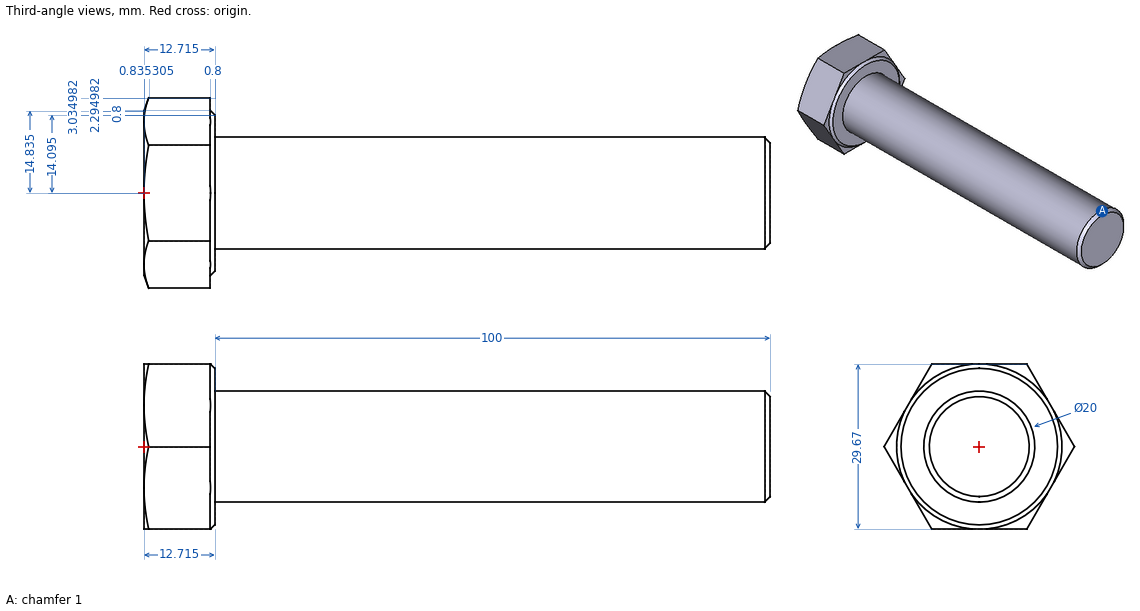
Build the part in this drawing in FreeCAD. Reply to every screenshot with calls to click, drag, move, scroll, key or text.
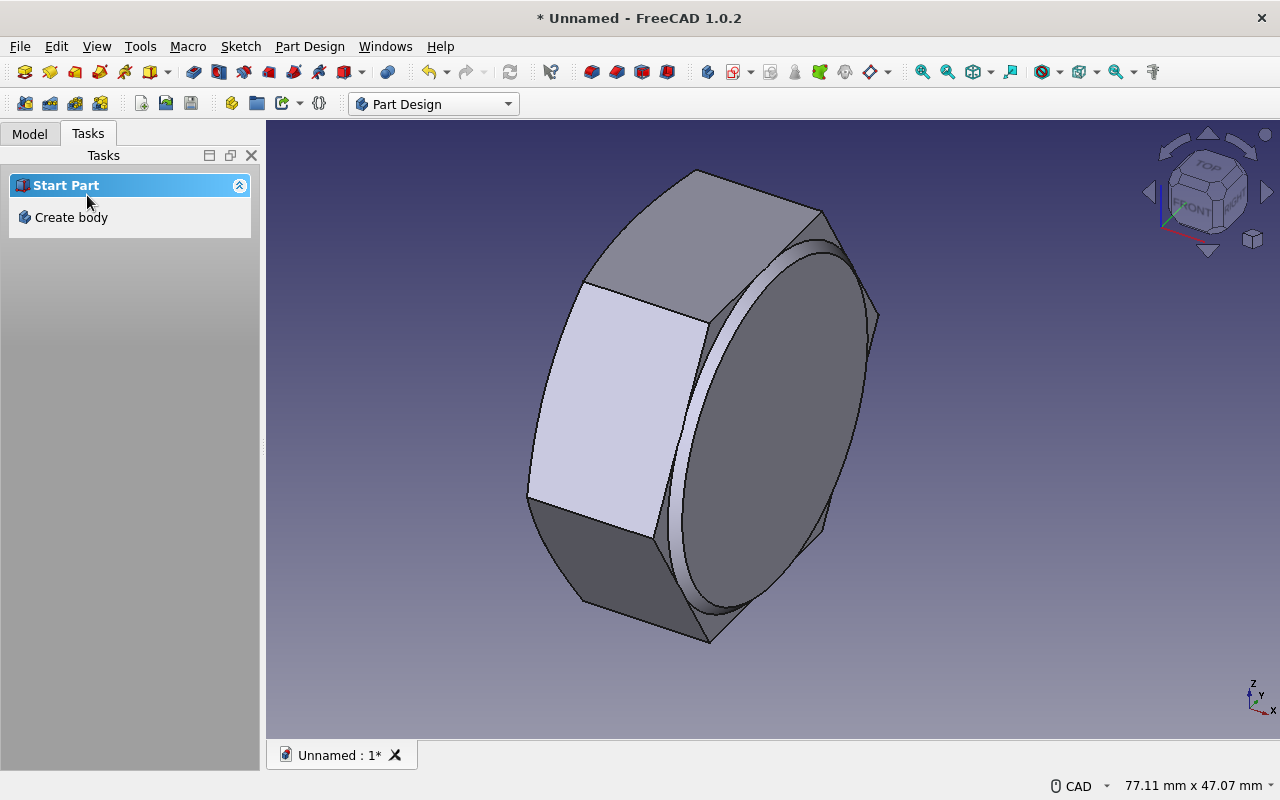
key(v)
key(f)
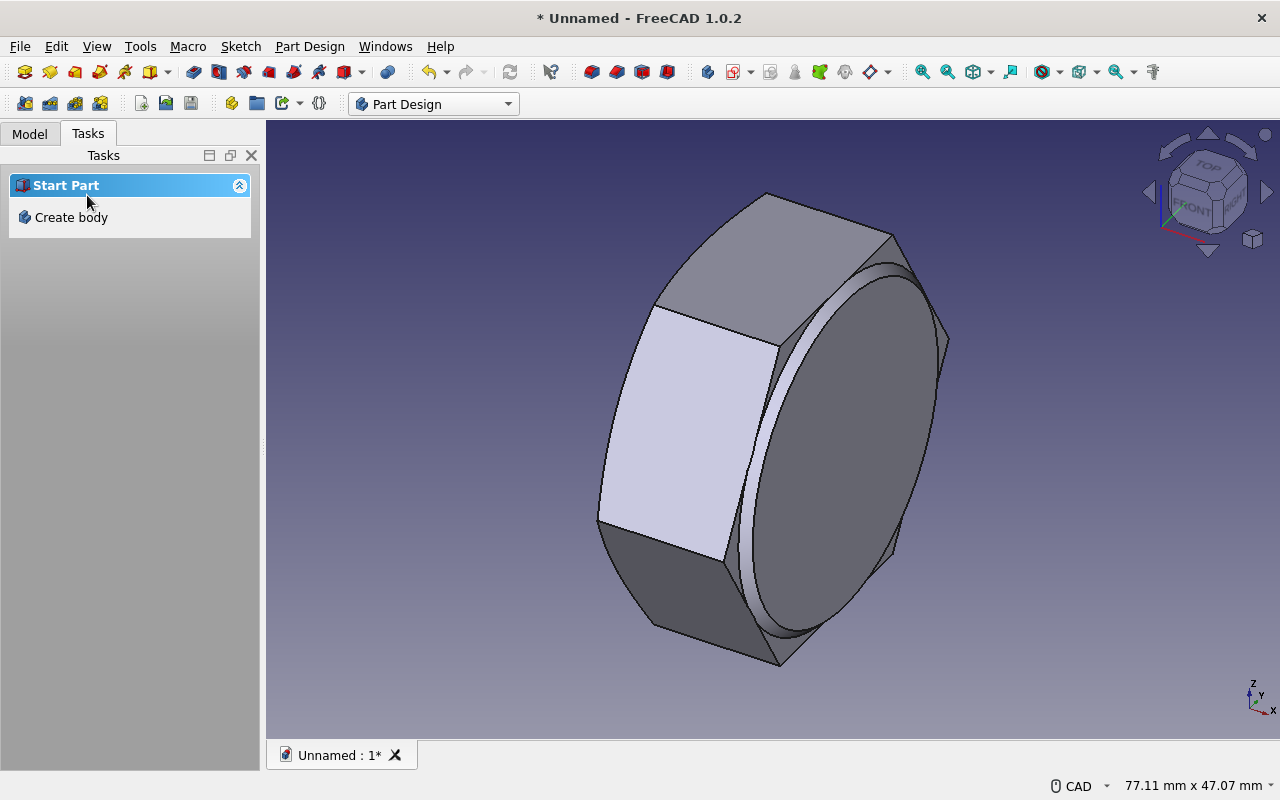
click(845, 452)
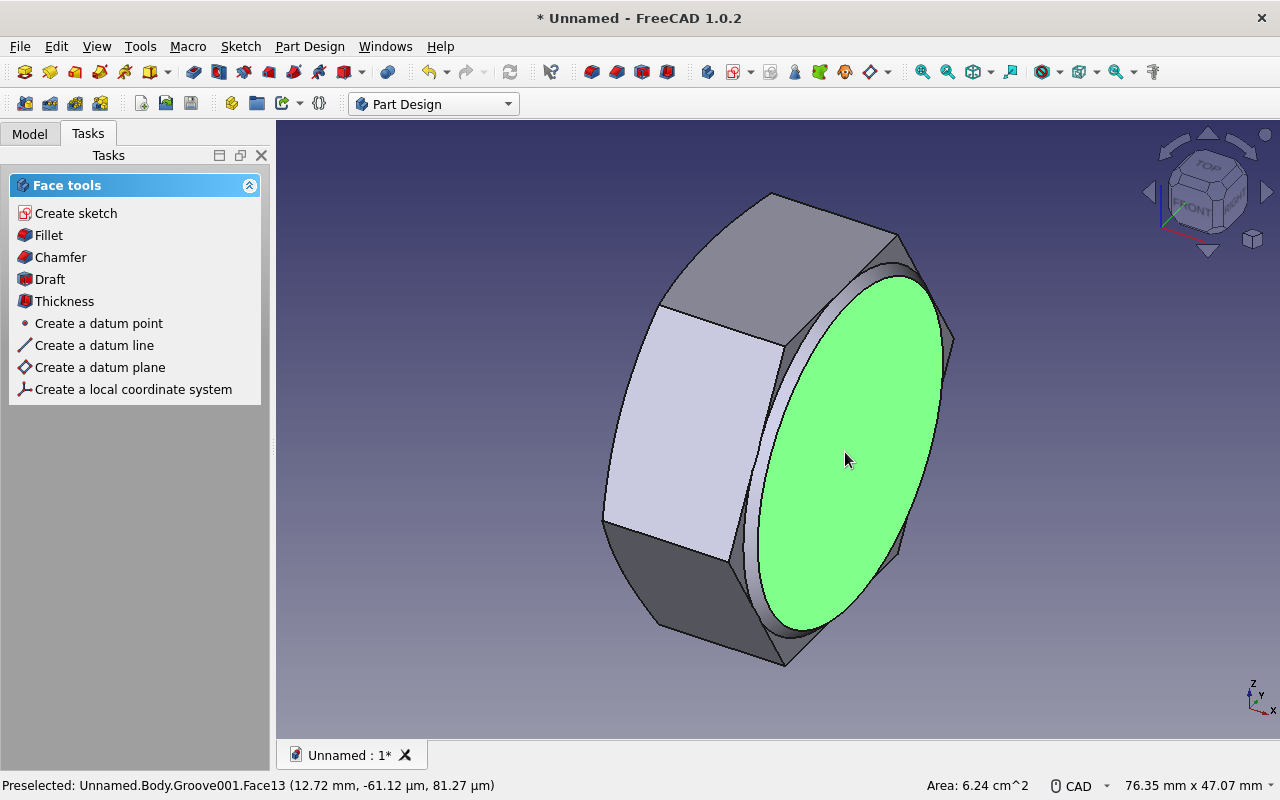
click(732, 72)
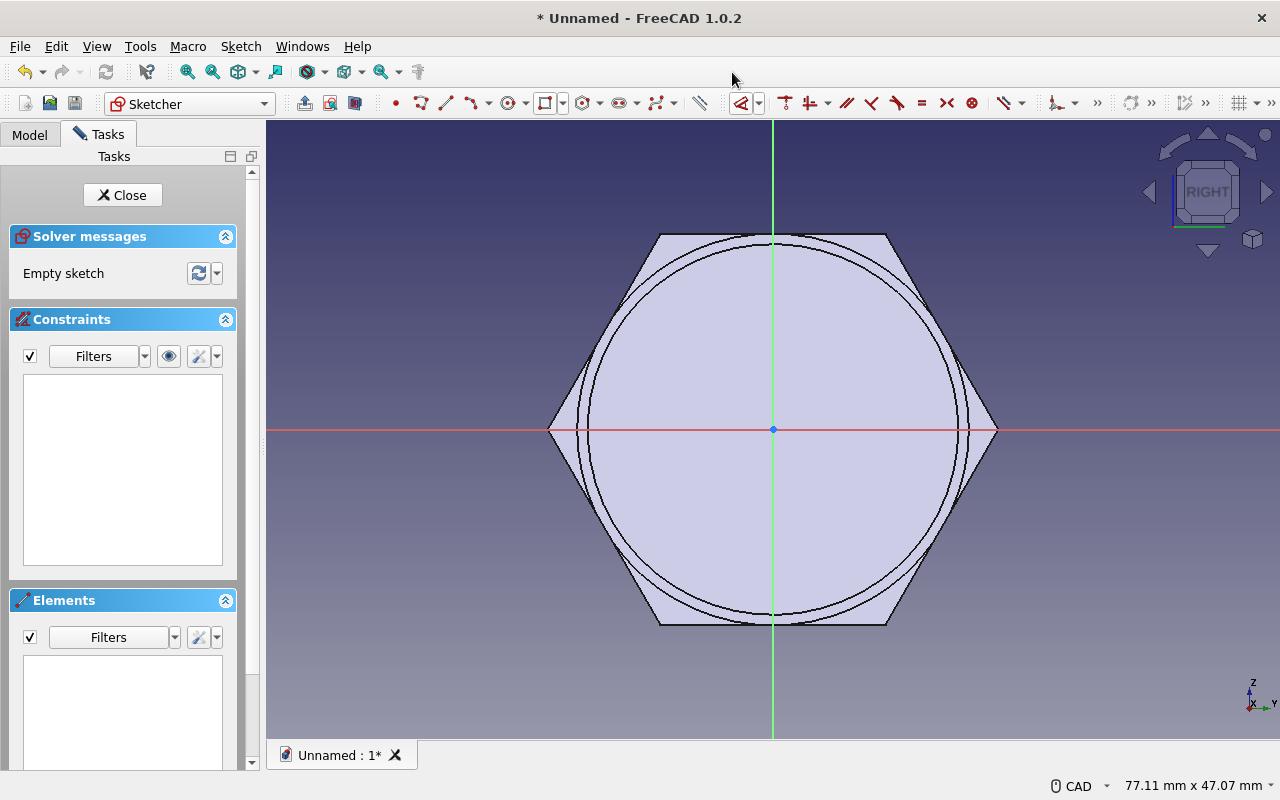
scroll(912, 429, up, 2)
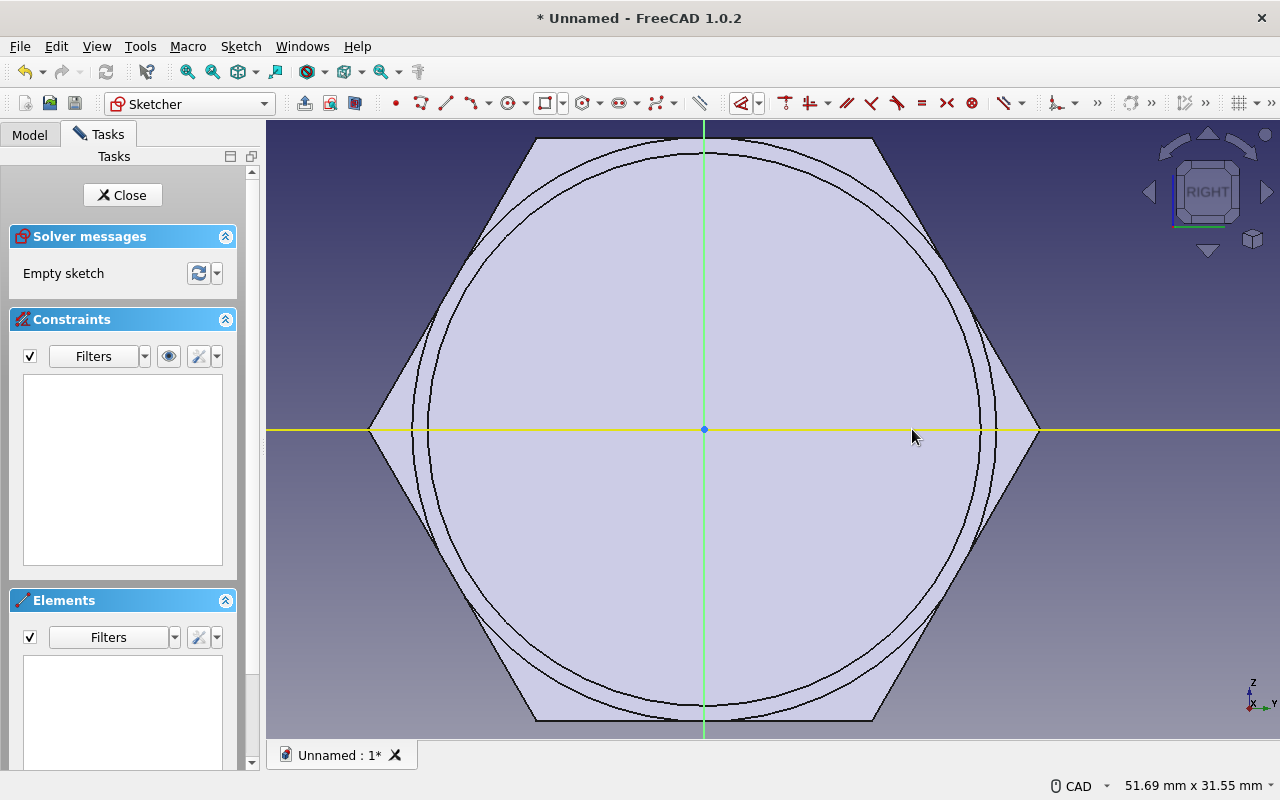
key(g)
key(c)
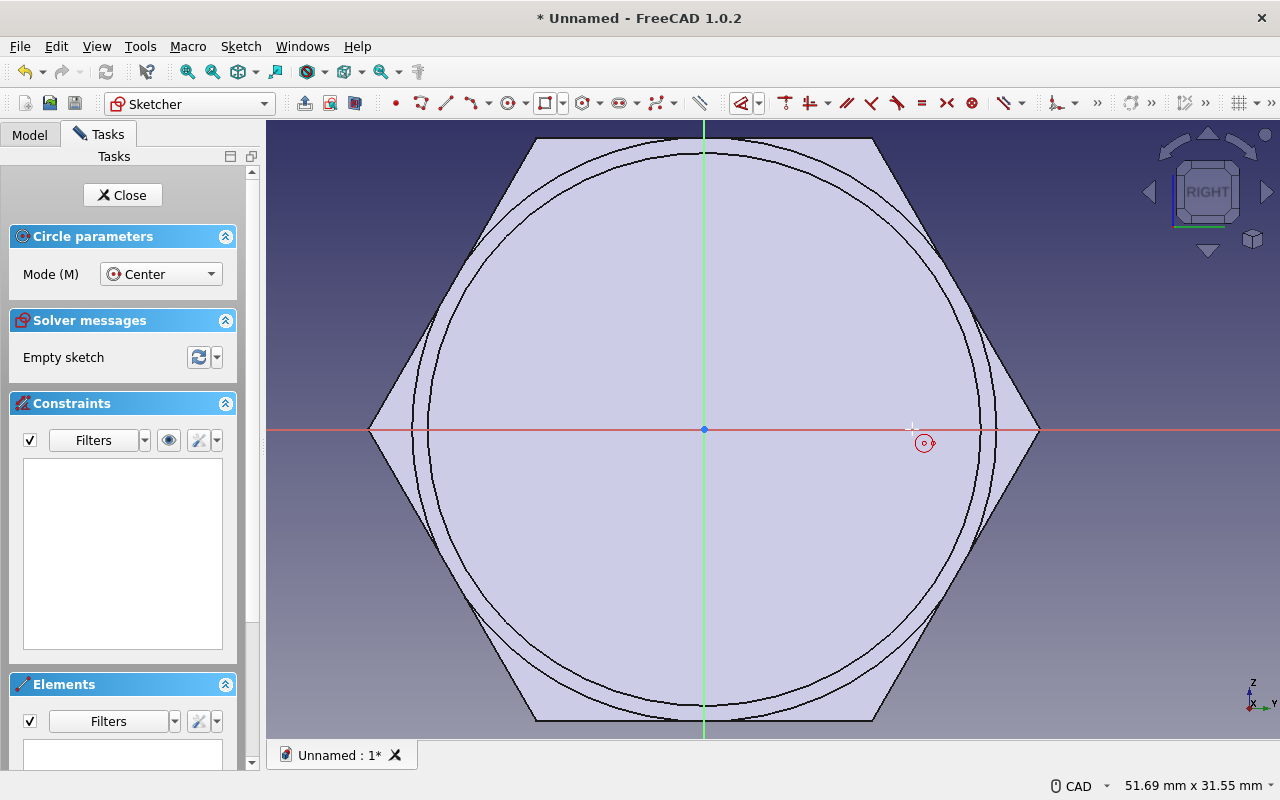
click(704, 429)
move(843, 291)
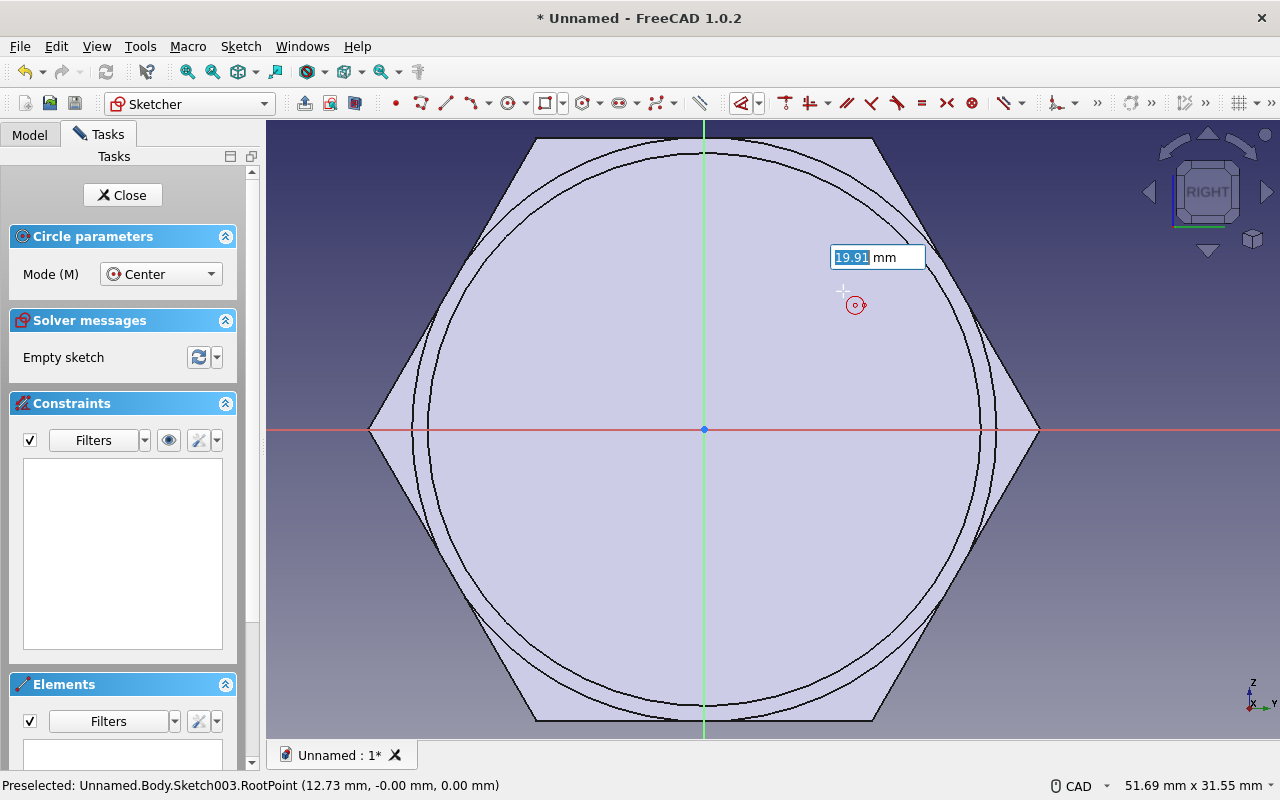
text(20)
key(Return)
key(Escape)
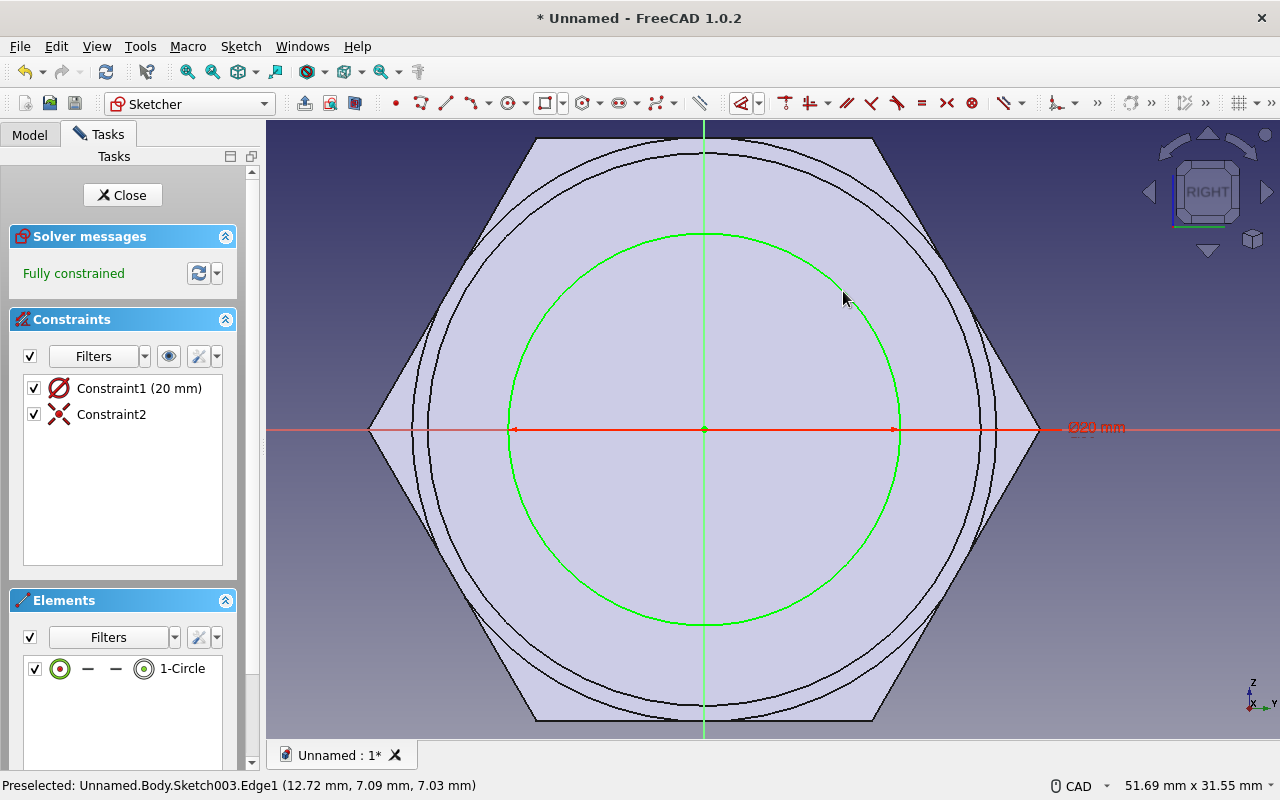
click(123, 195)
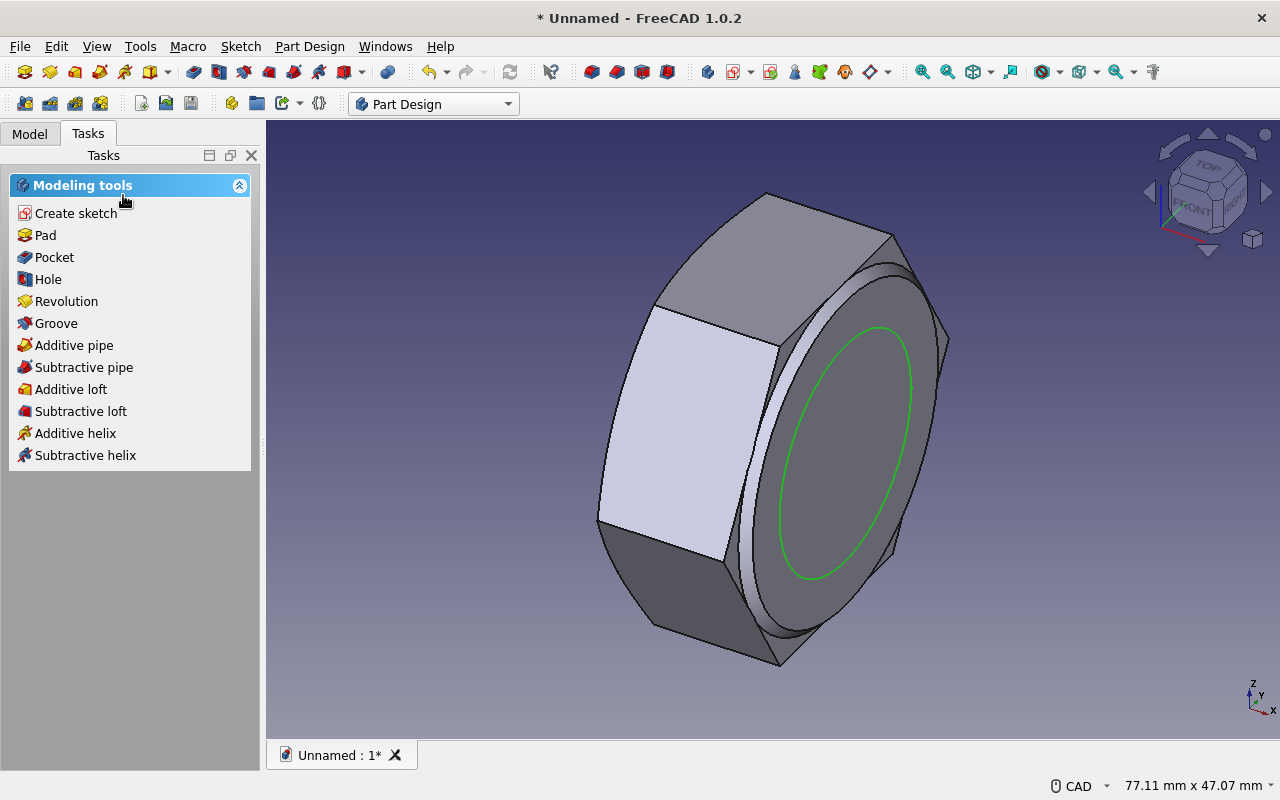
click(25, 72)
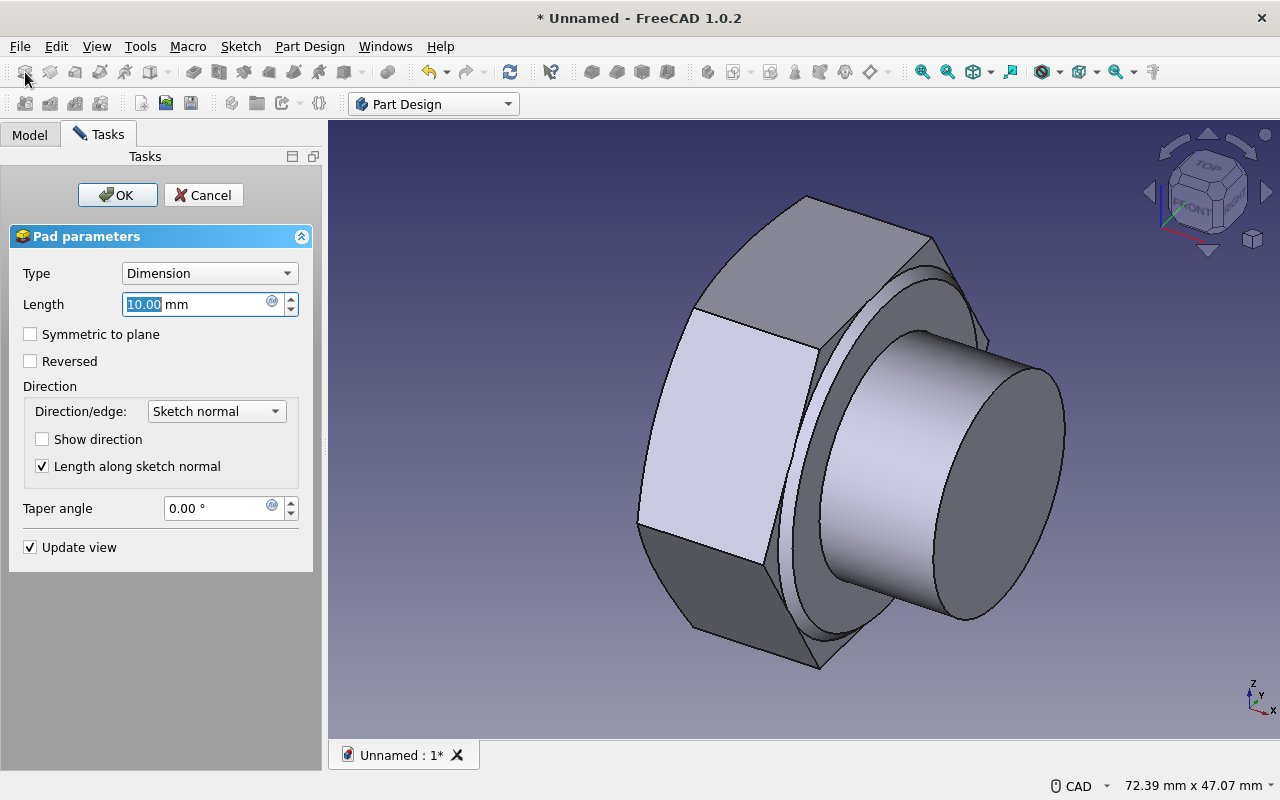
text(100)
key(Tab)